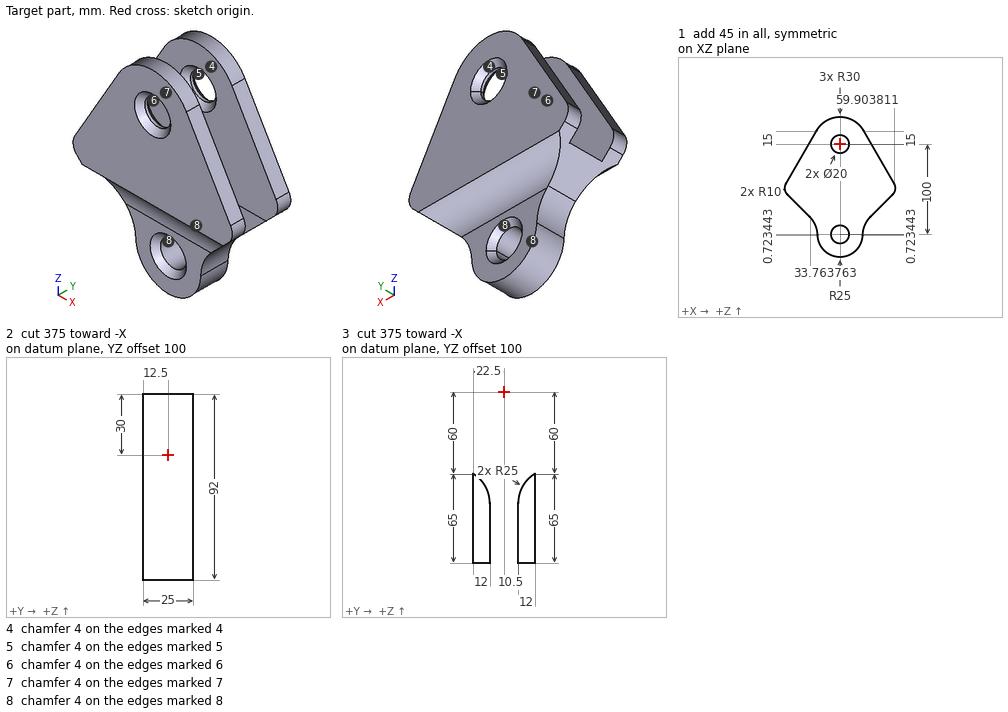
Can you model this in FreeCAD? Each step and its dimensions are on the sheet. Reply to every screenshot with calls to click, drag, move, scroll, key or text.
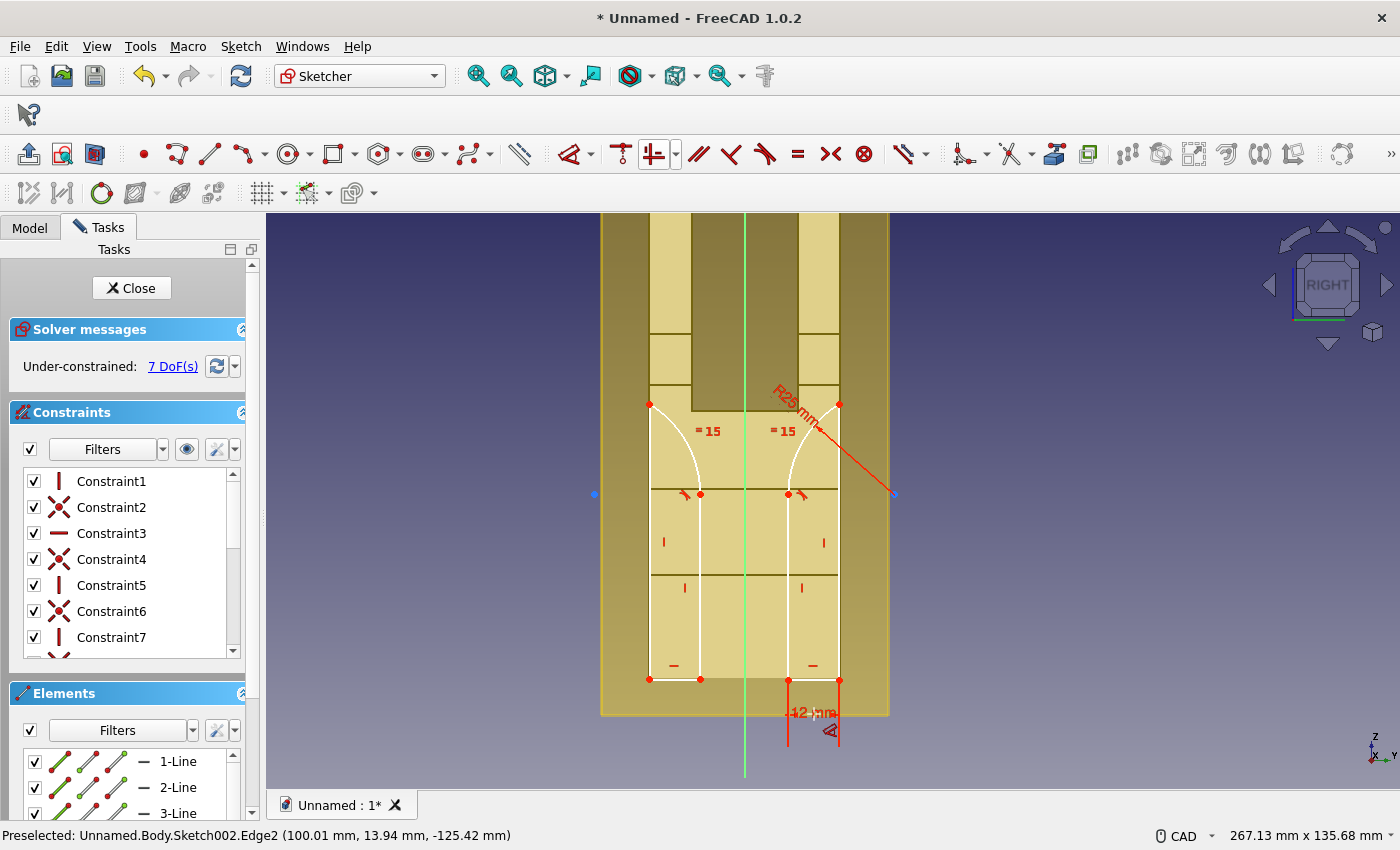
click(839, 597)
click(873, 542)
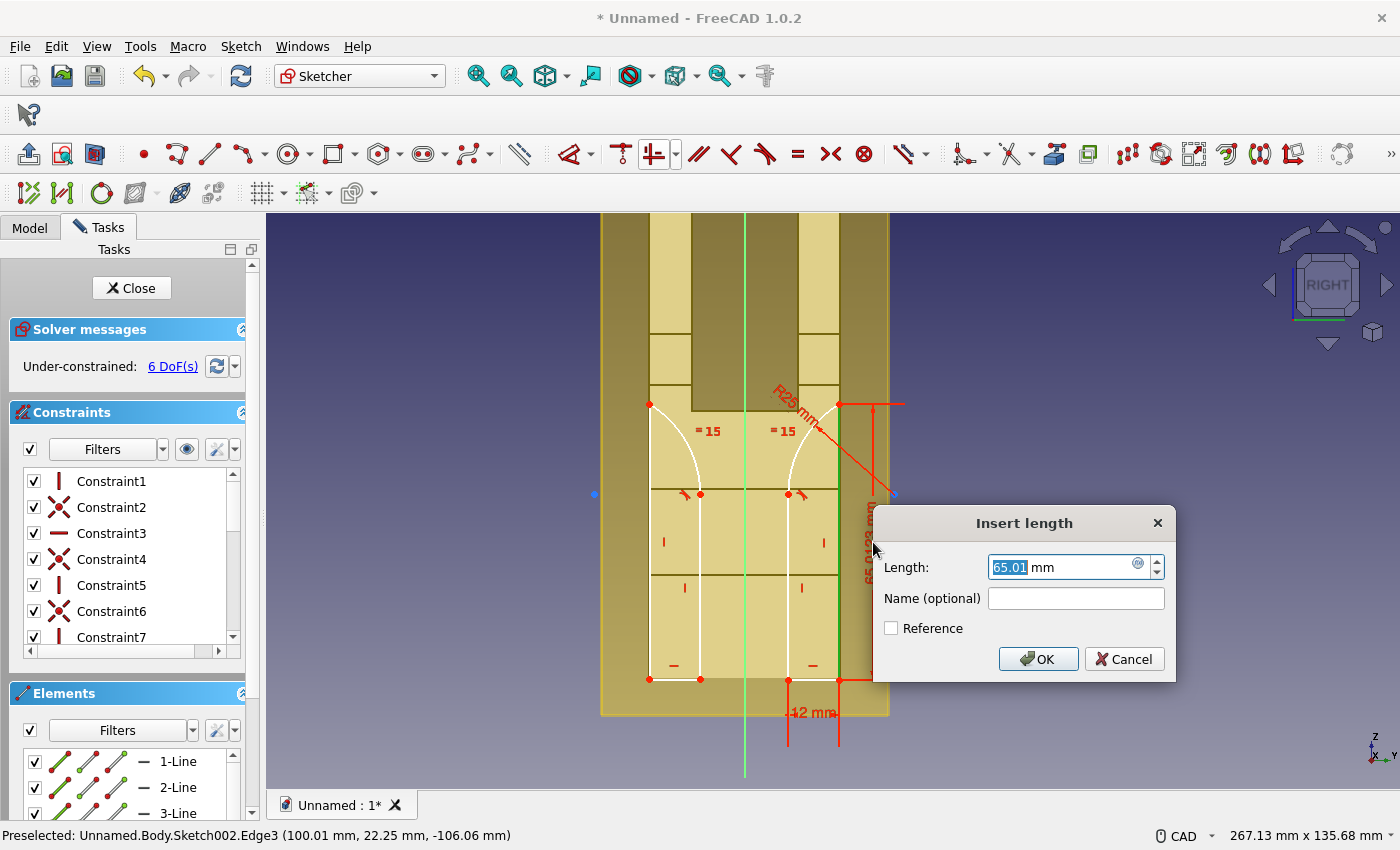
text(65)
key(Return)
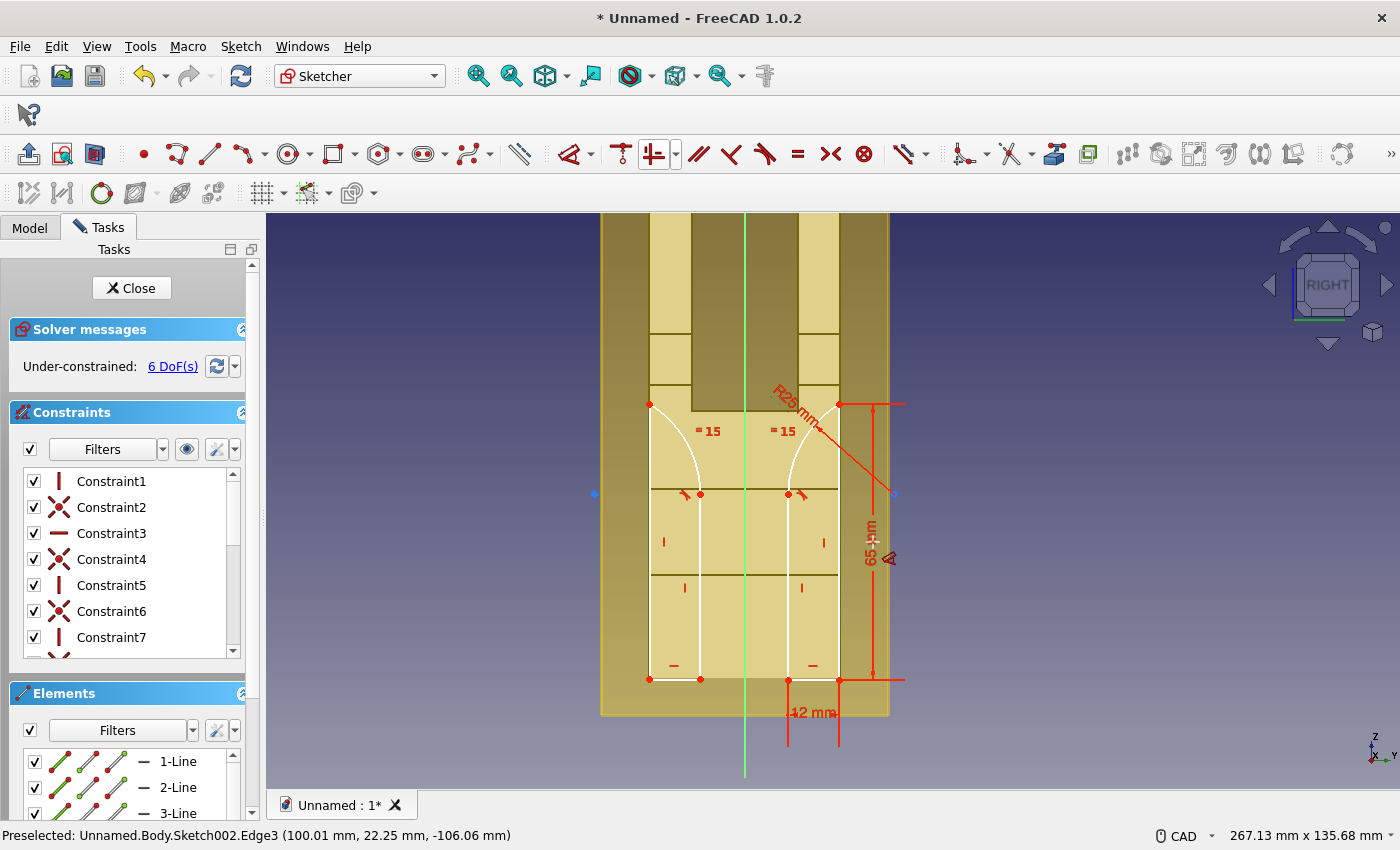
click(650, 487)
click(616, 542)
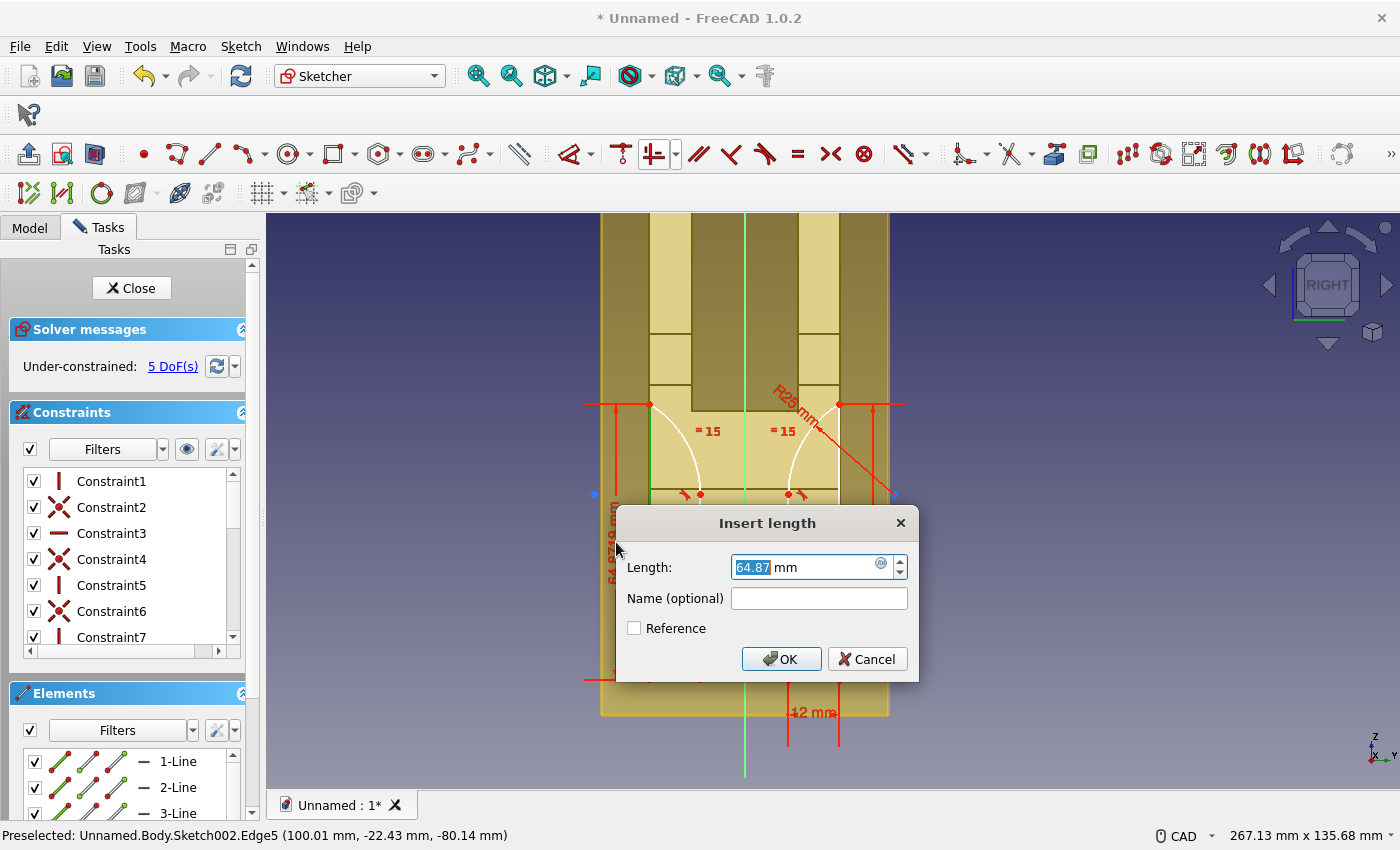
text(65)
key(Return)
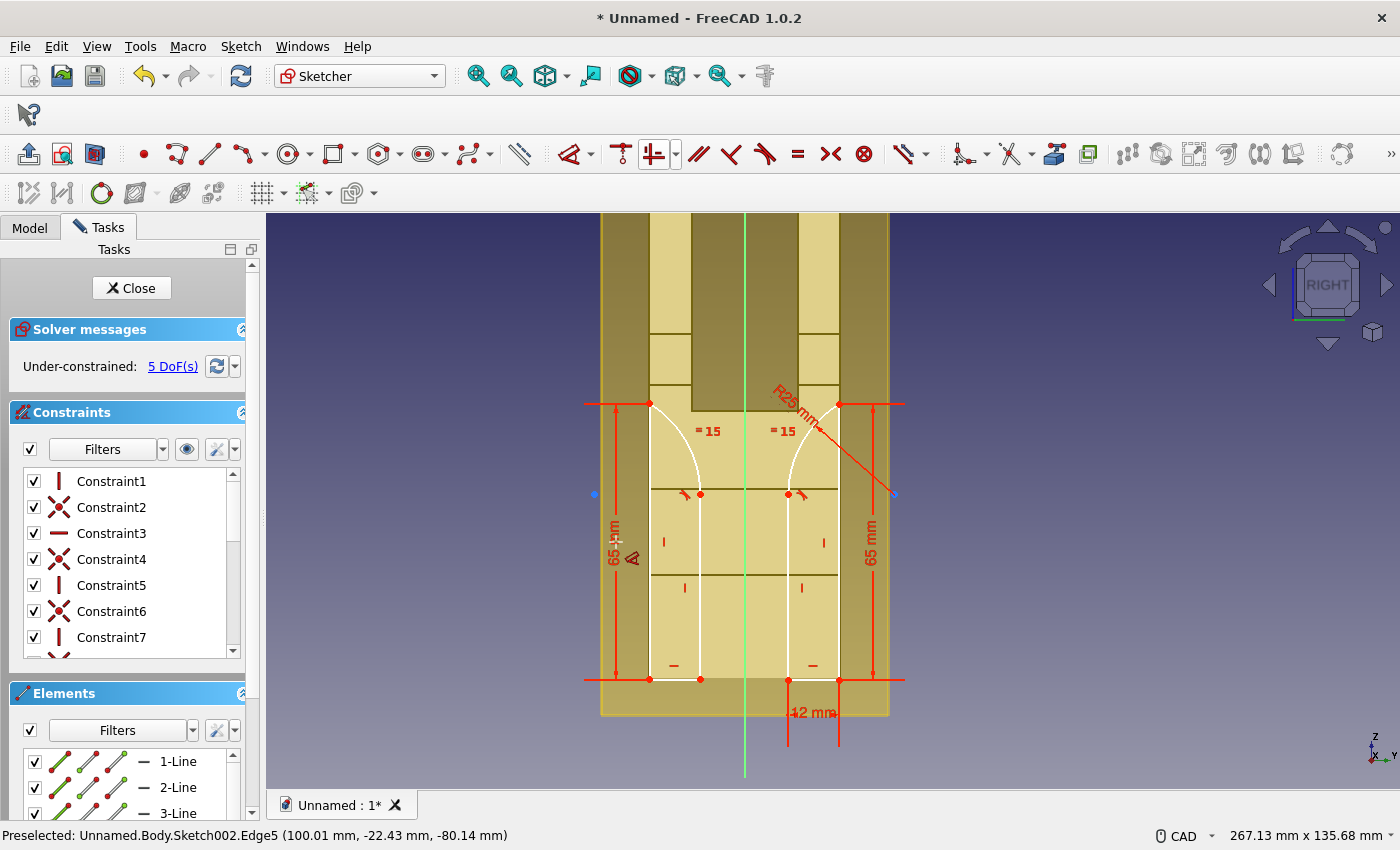
click(665, 680)
click(675, 714)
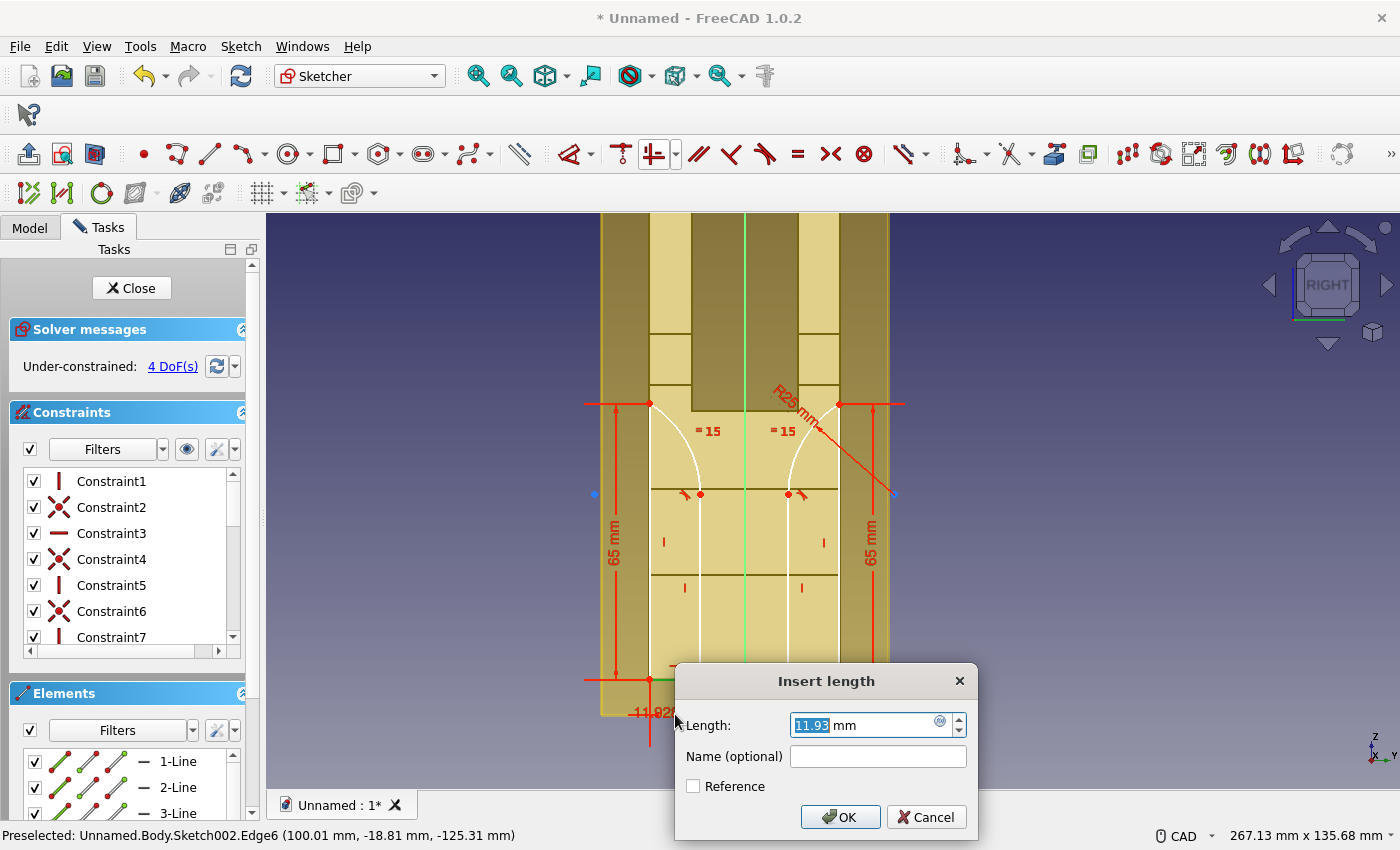
text(12)
key(Return)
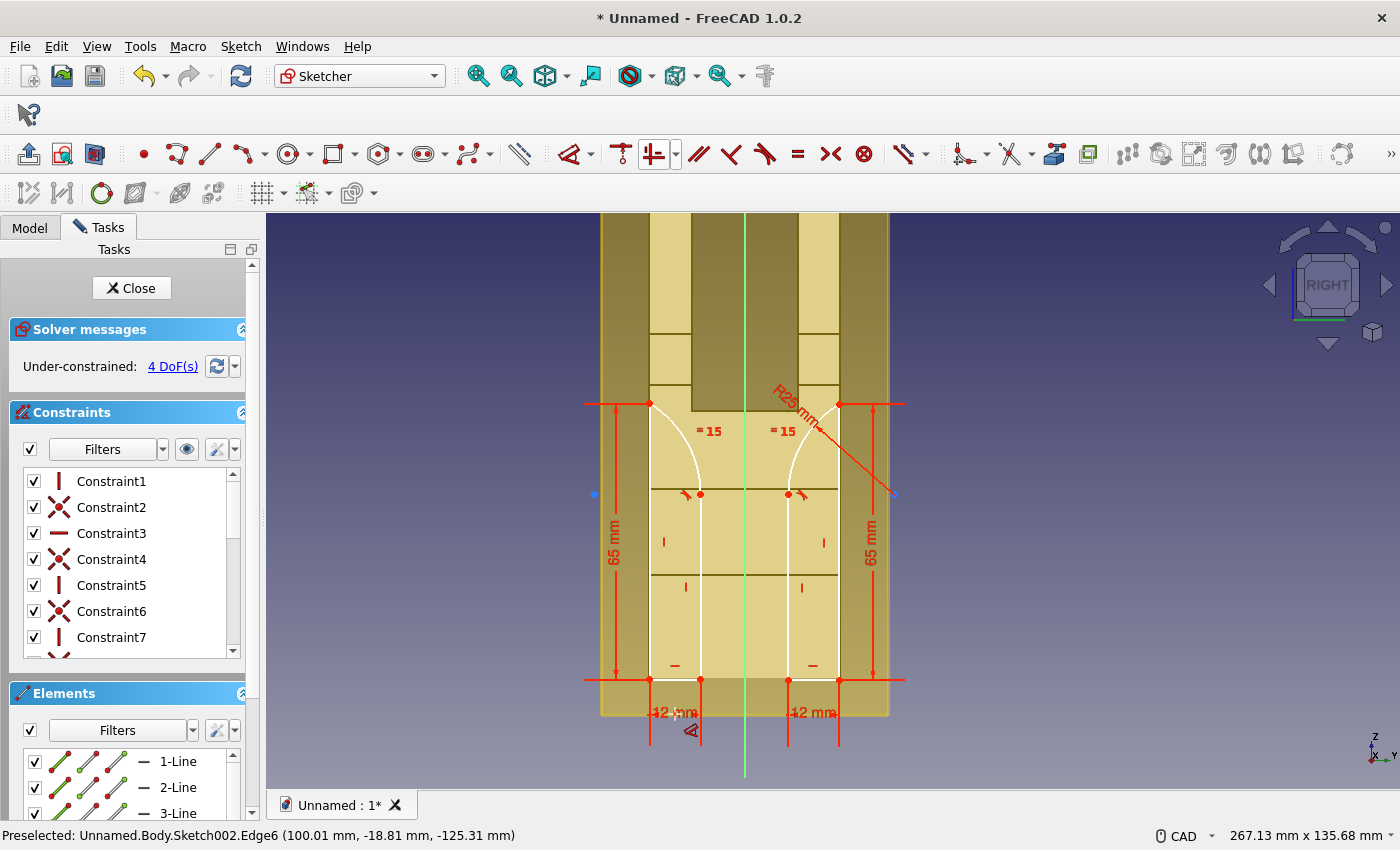
click(839, 404)
click(873, 323)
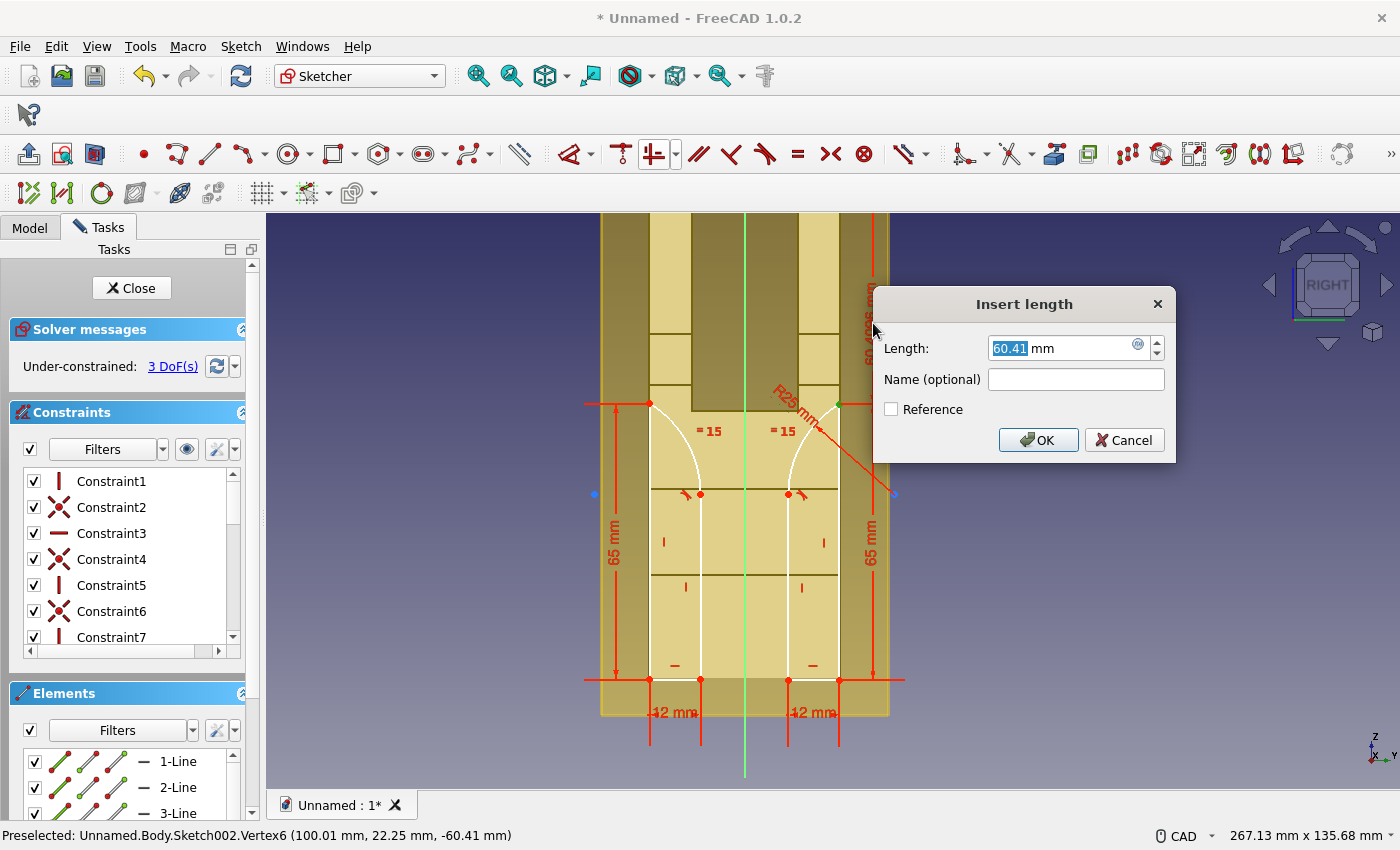
text(60)
key(Return)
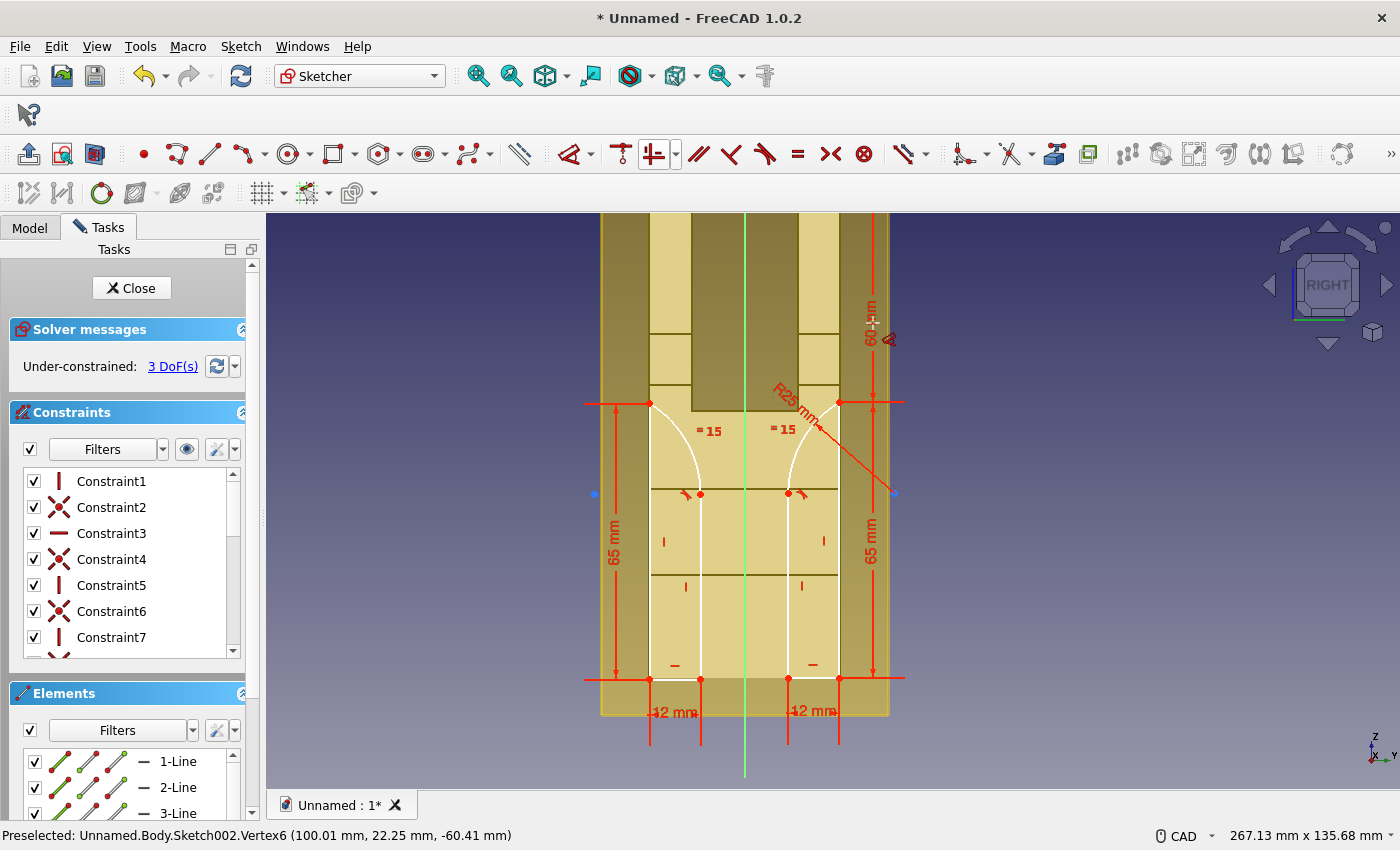
click(650, 404)
click(616, 322)